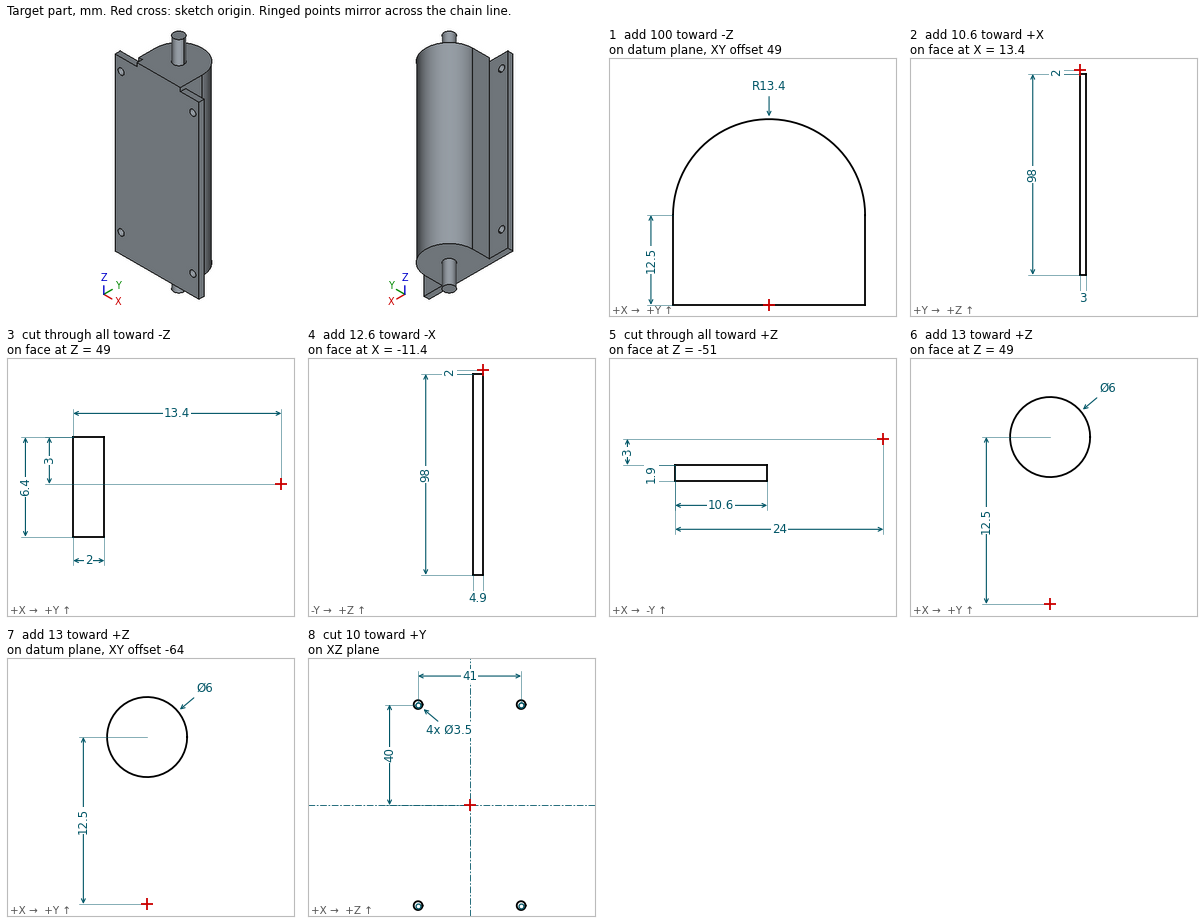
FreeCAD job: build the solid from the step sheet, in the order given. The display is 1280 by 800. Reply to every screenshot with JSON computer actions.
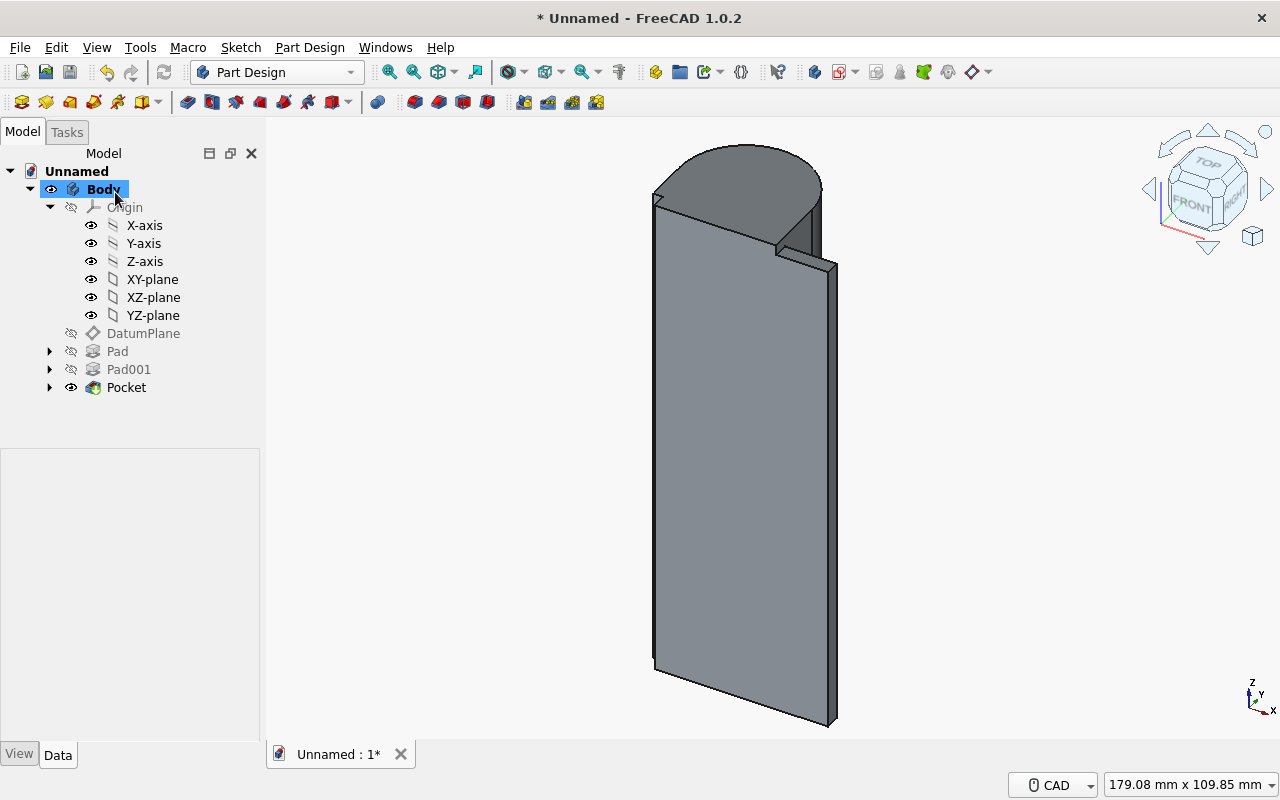
{"action": "key", "text": "6"}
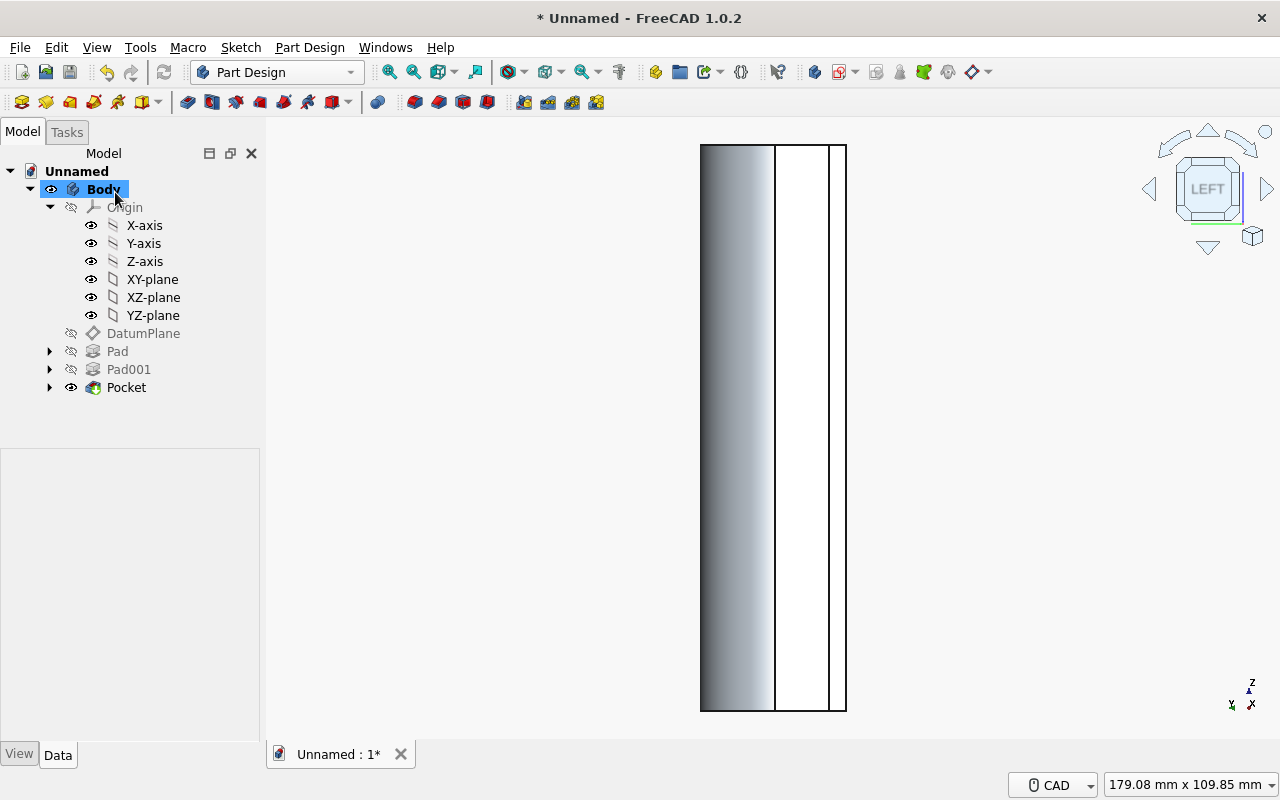
{"action": "left_click", "coordinate": [838, 184]}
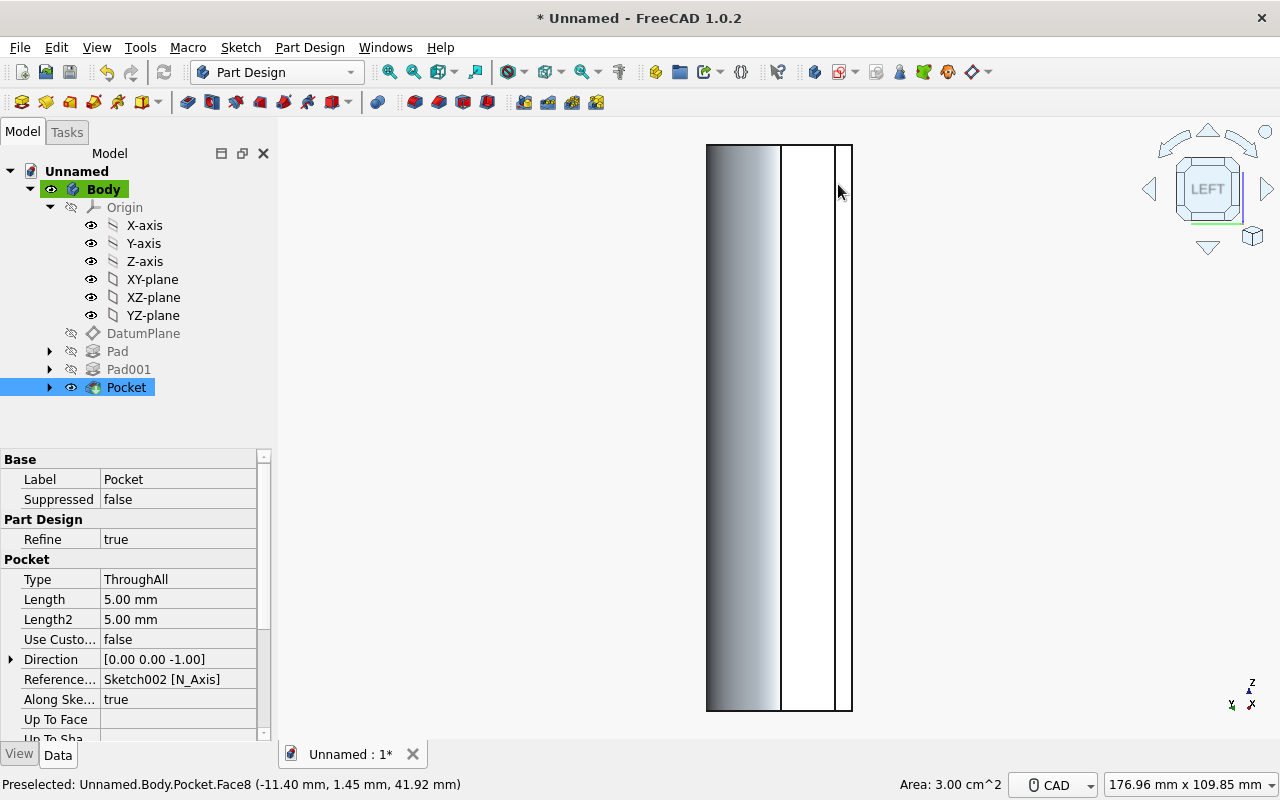
{"action": "left_click", "coordinate": [840, 72]}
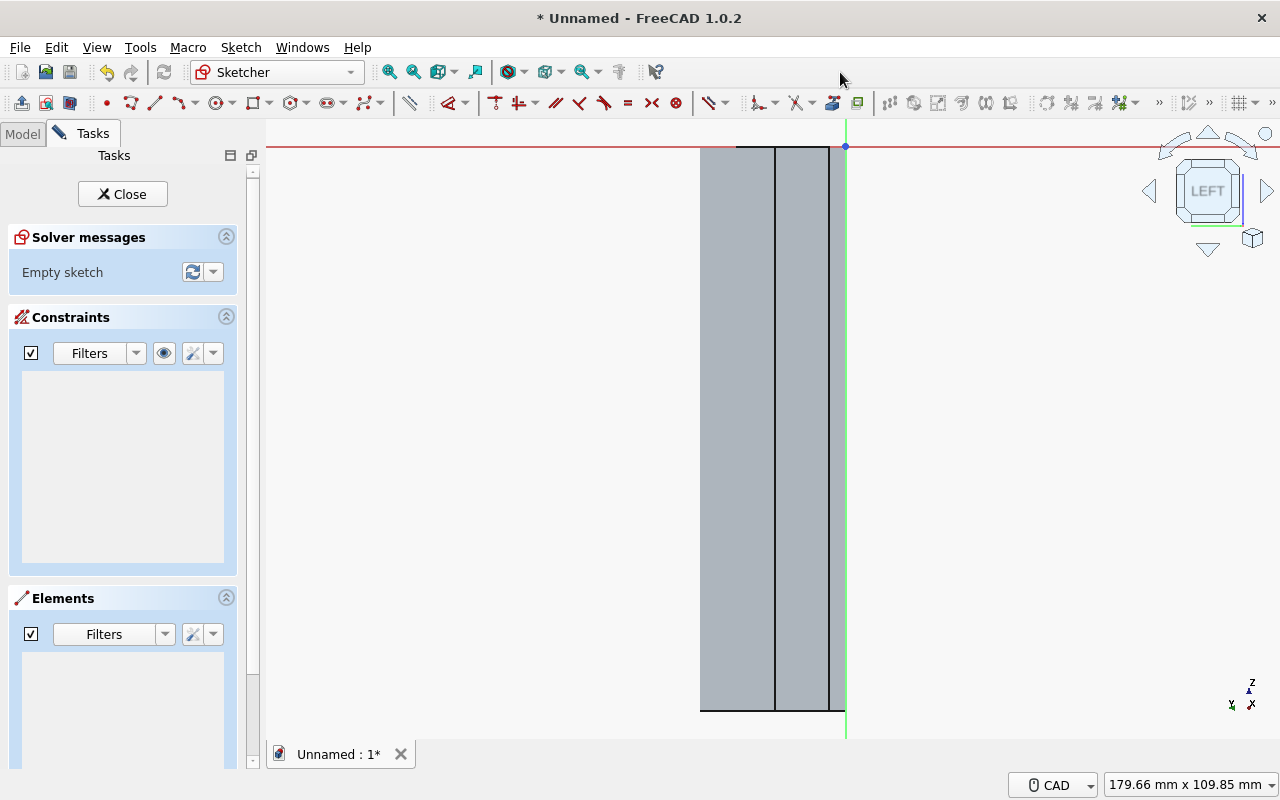
{"action": "left_click", "coordinate": [70, 104]}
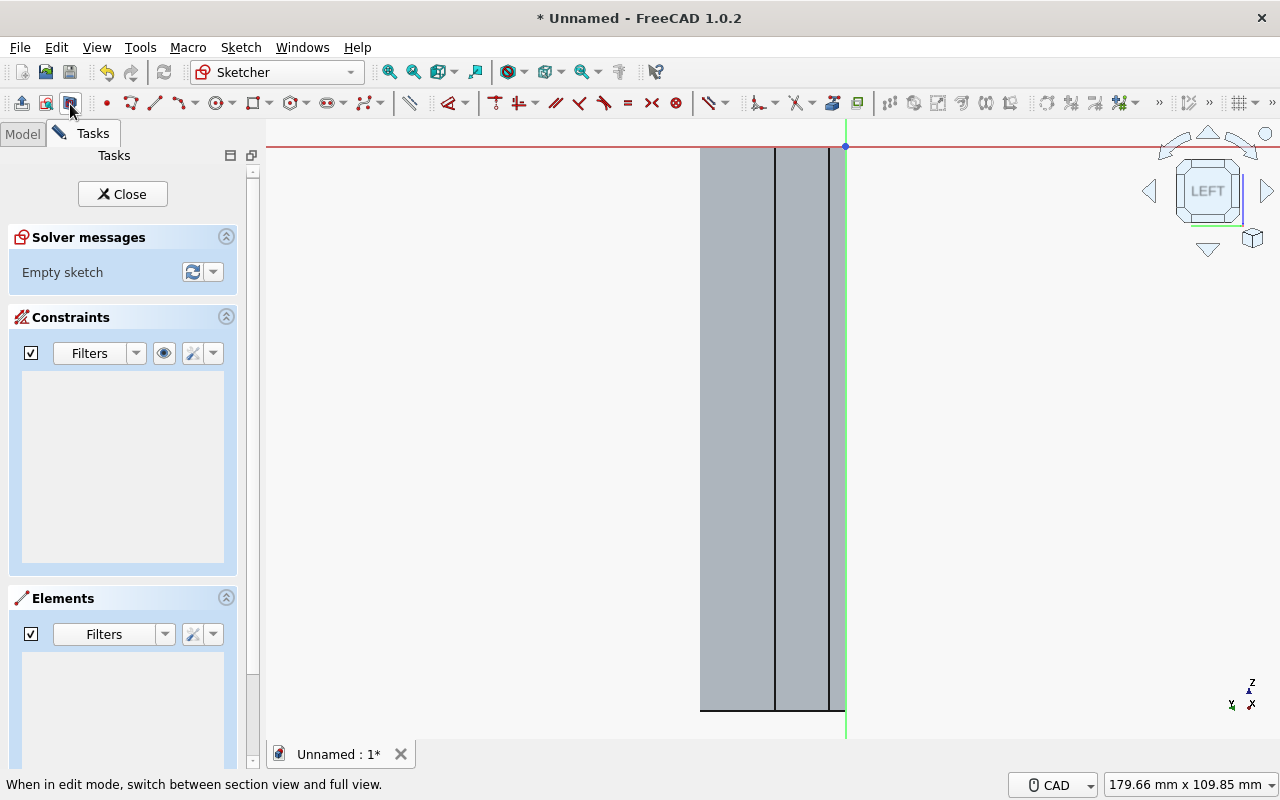
{"action": "scroll", "coordinate": [445, 429], "scroll_direction": "down", "scroll_amount": 2}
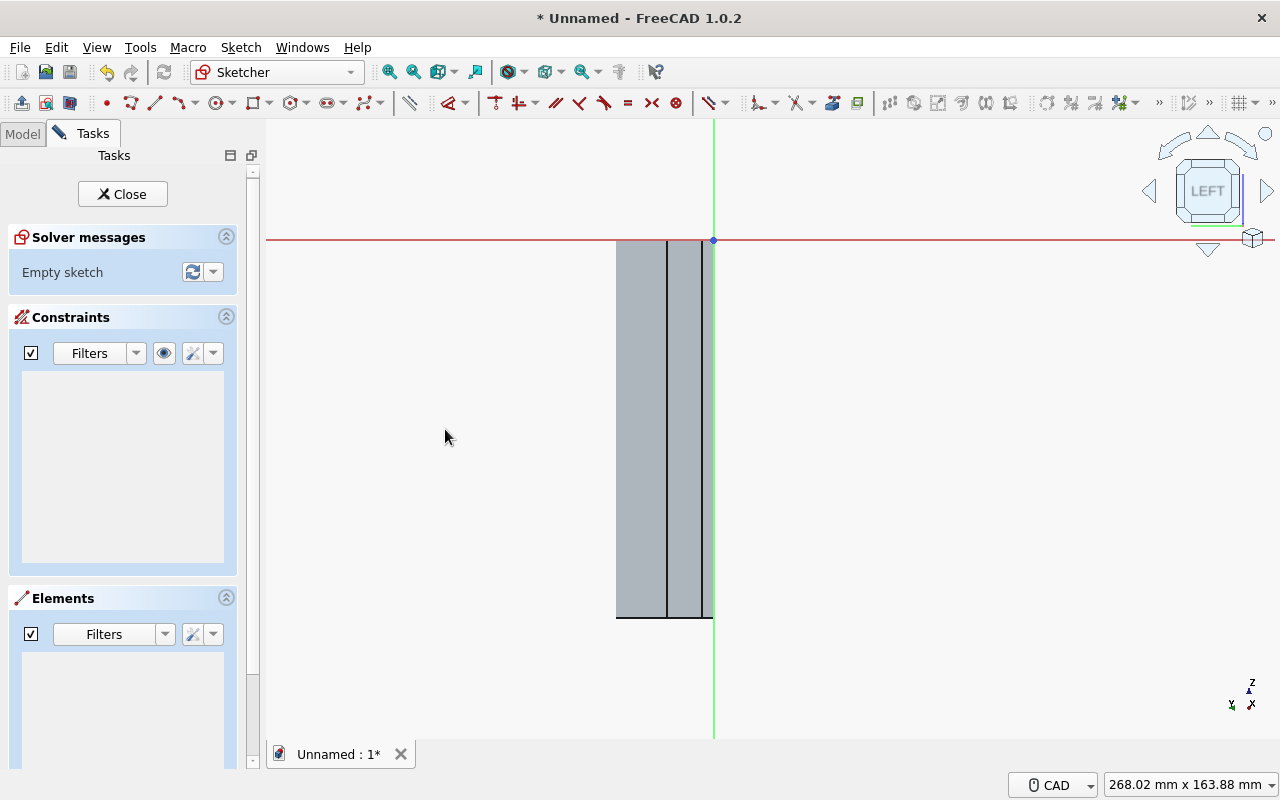
{"action": "left_click", "coordinate": [254, 104]}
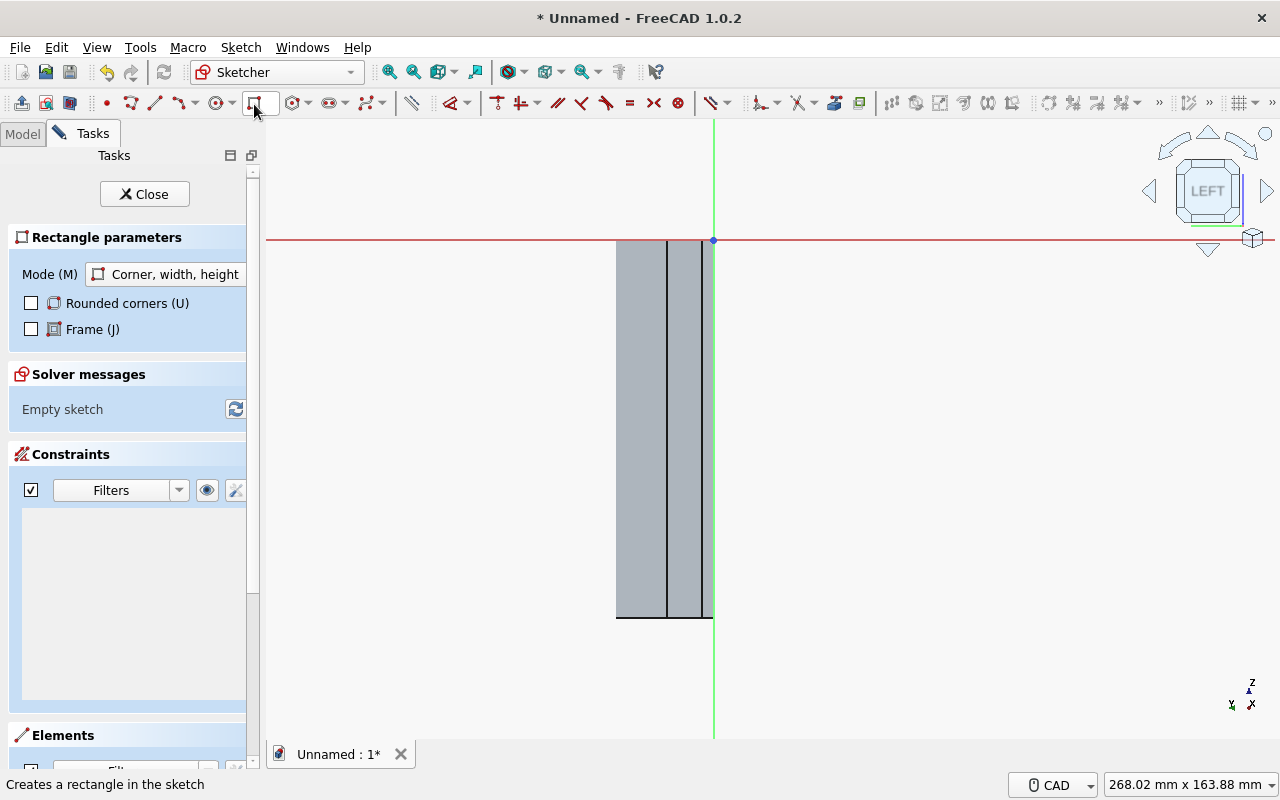
{"action": "scroll", "coordinate": [695, 248], "scroll_direction": "up", "scroll_amount": 4}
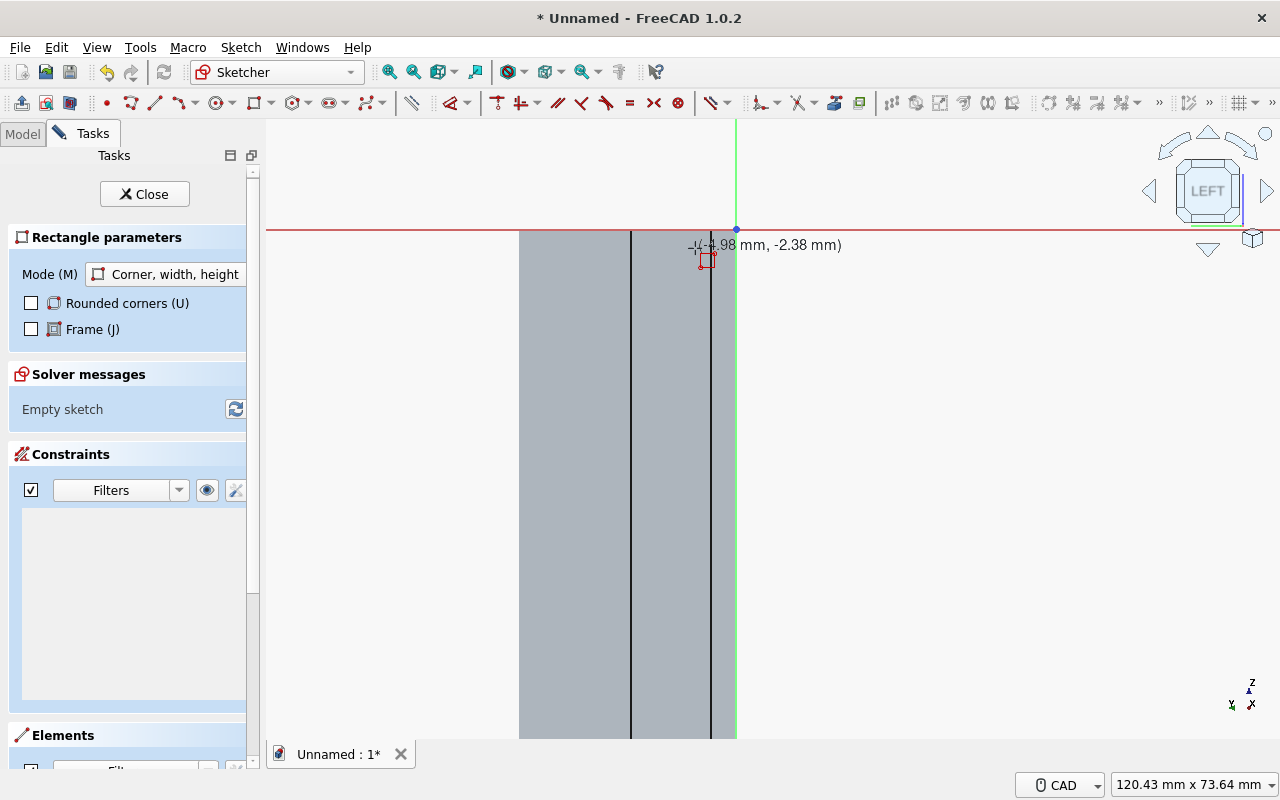
{"action": "left_click", "coordinate": [695, 247]}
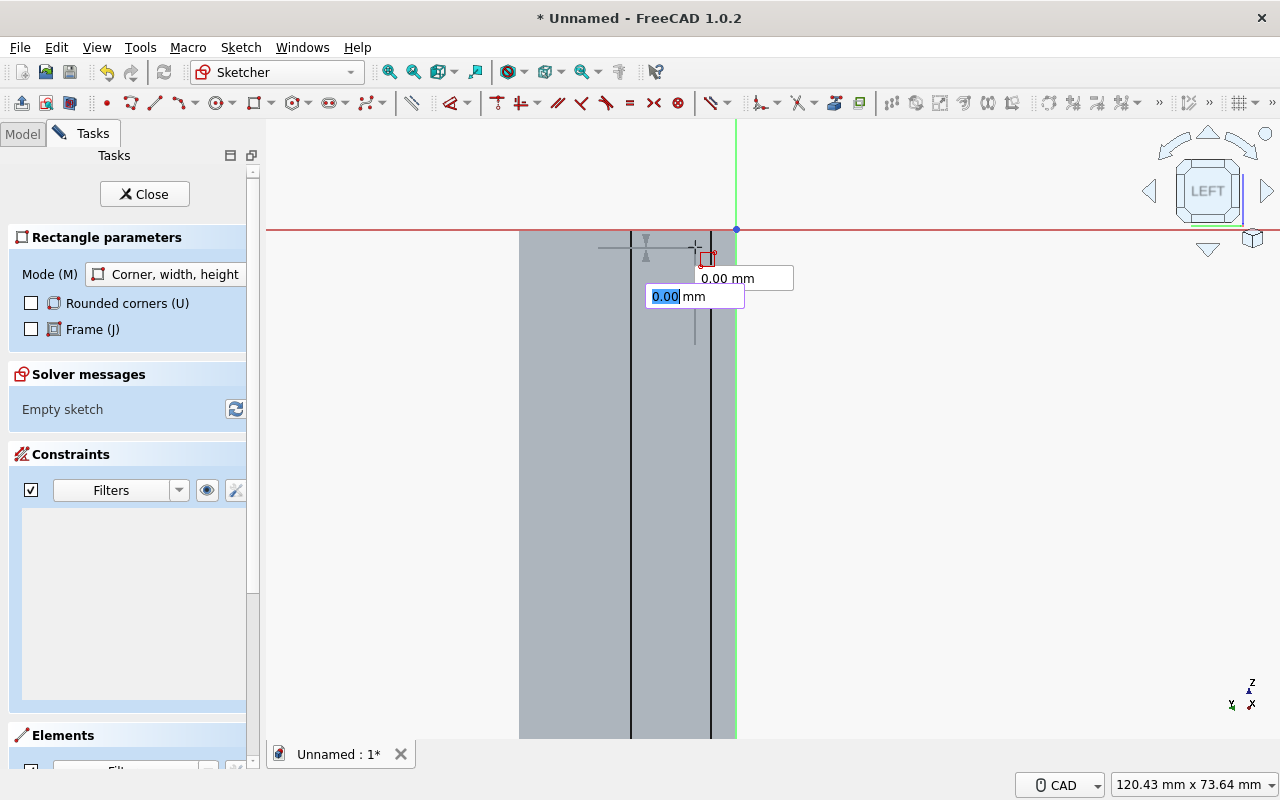
{"action": "scroll", "coordinate": [695, 248], "scroll_direction": "down", "scroll_amount": 4}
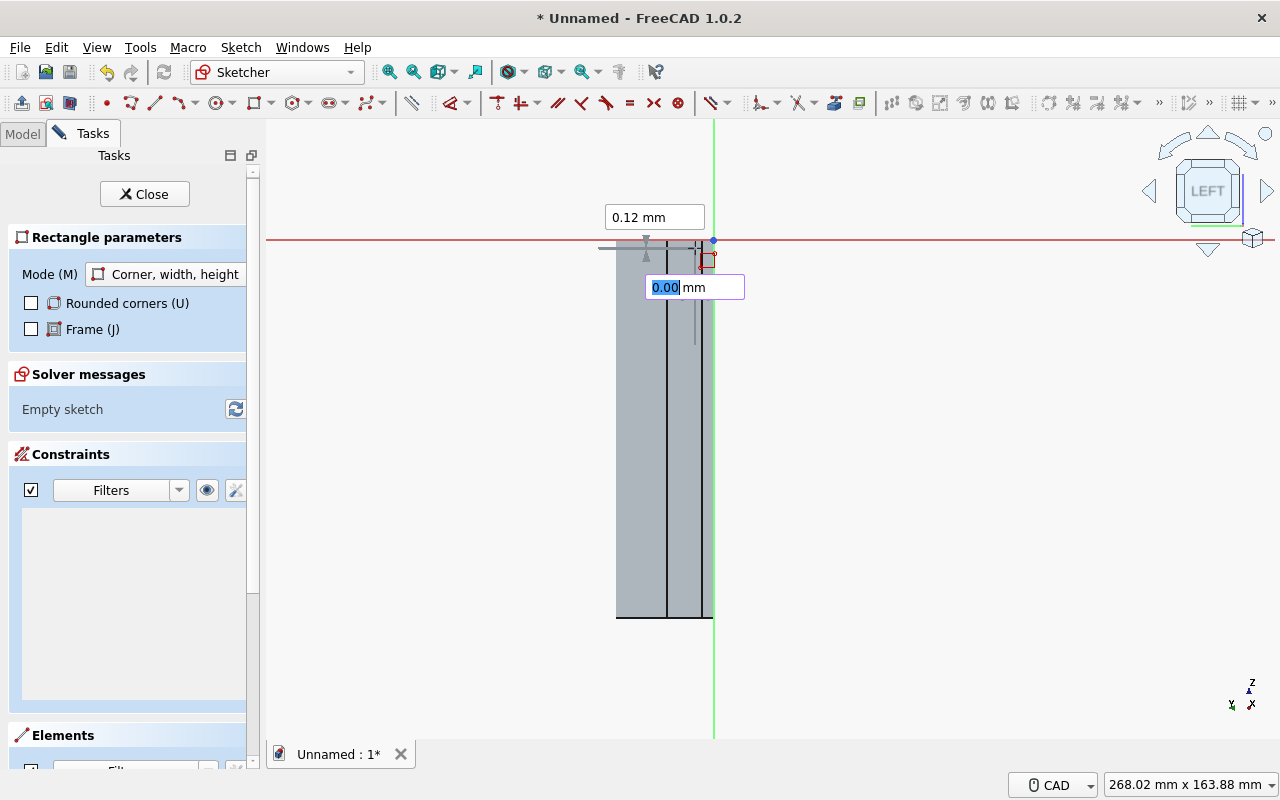
{"action": "left_click", "coordinate": [714, 618]}
{"action": "key", "text": "Escape"}